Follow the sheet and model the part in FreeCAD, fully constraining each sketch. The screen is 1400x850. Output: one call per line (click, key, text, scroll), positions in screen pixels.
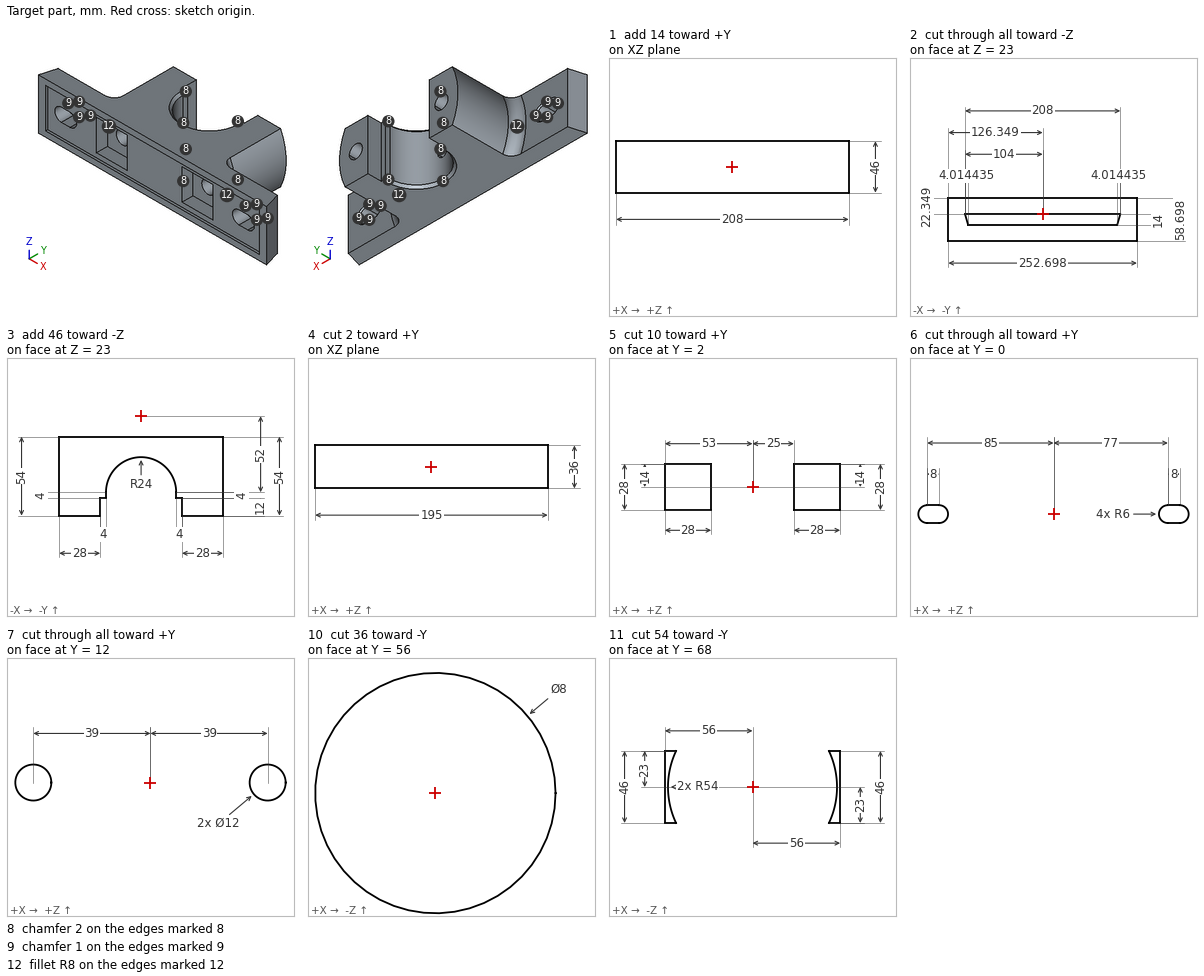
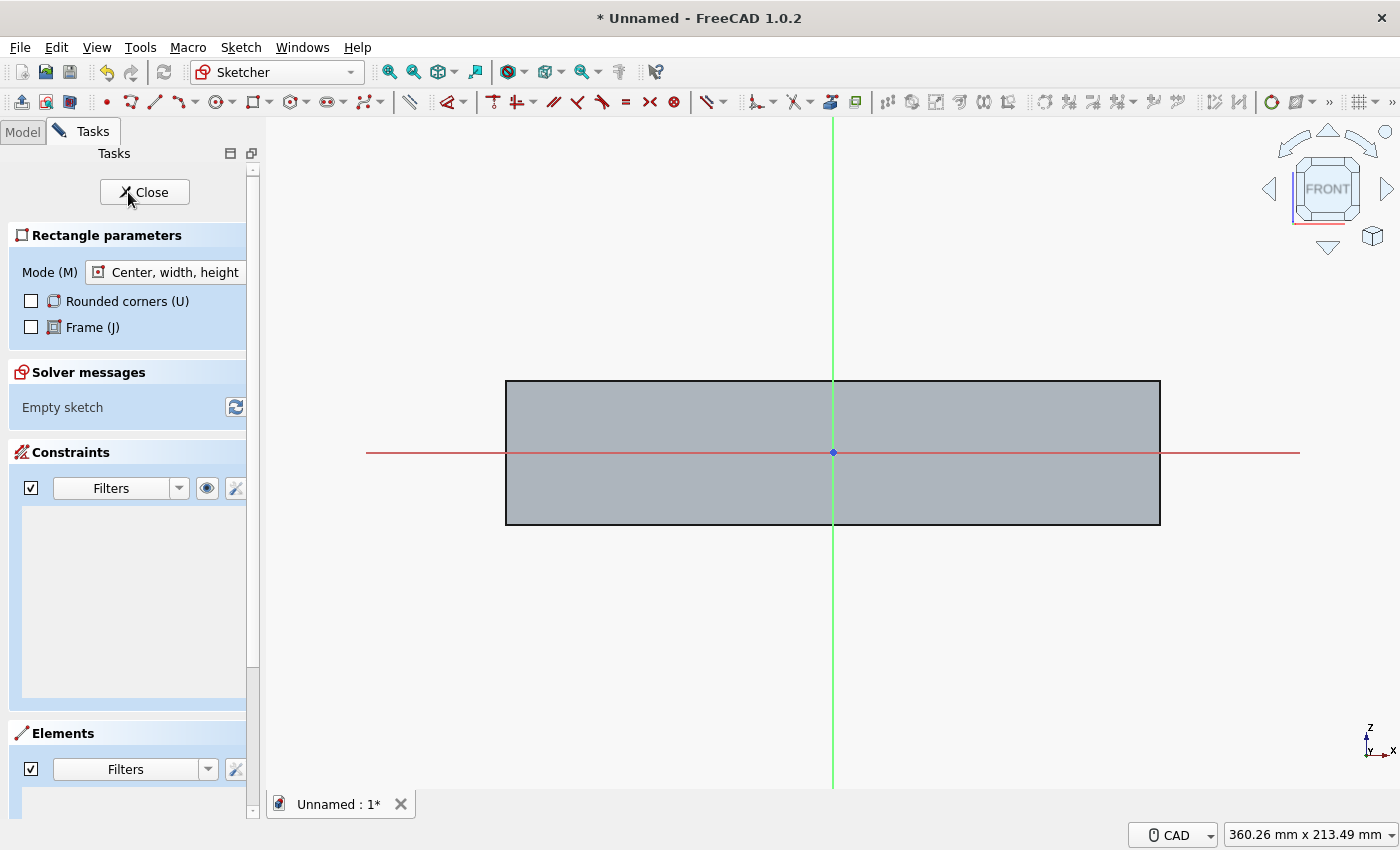
click(833, 453)
move(1140, 396)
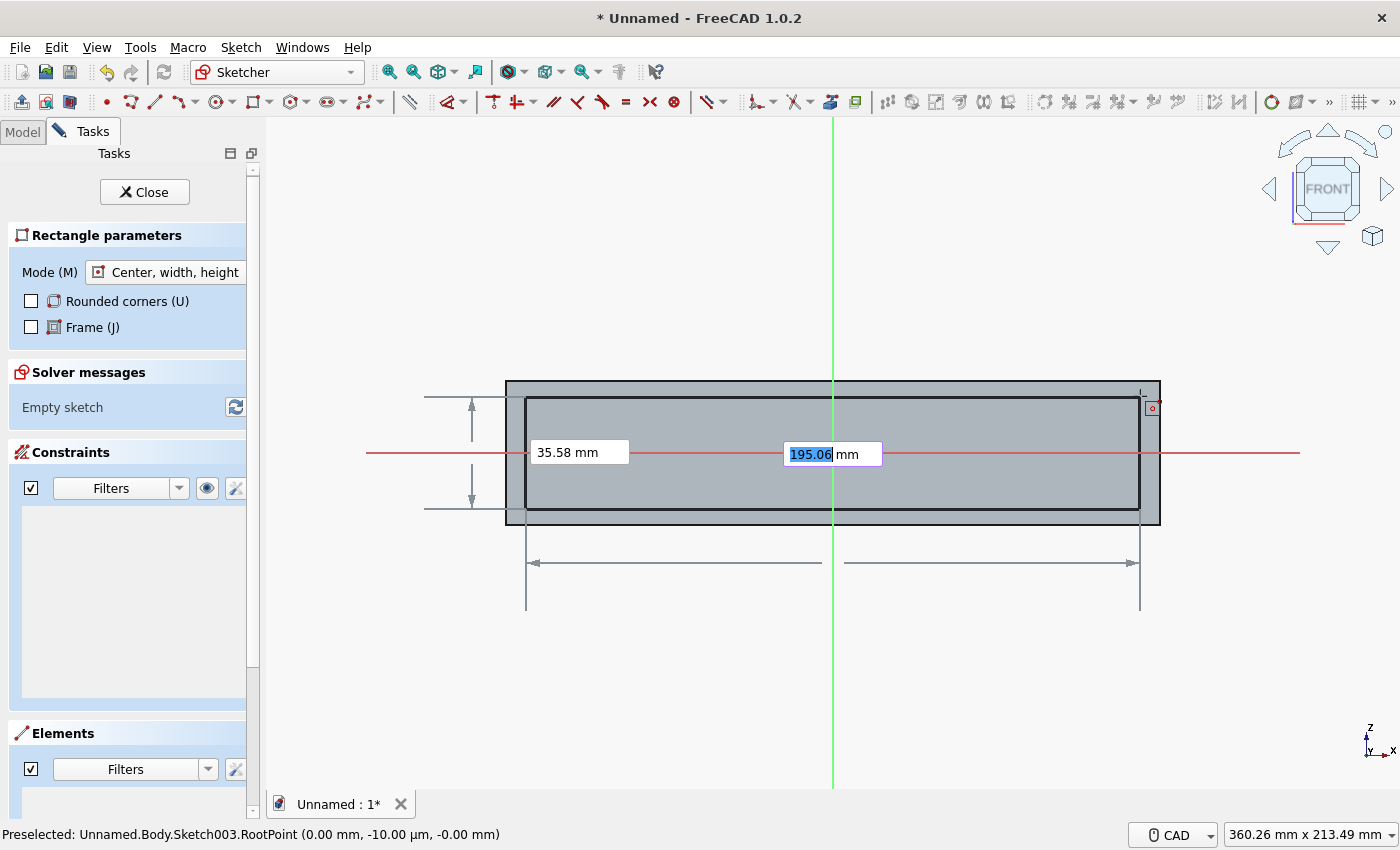
text(195)
key(Tab)
text(36)
key(Return)
key(Escape)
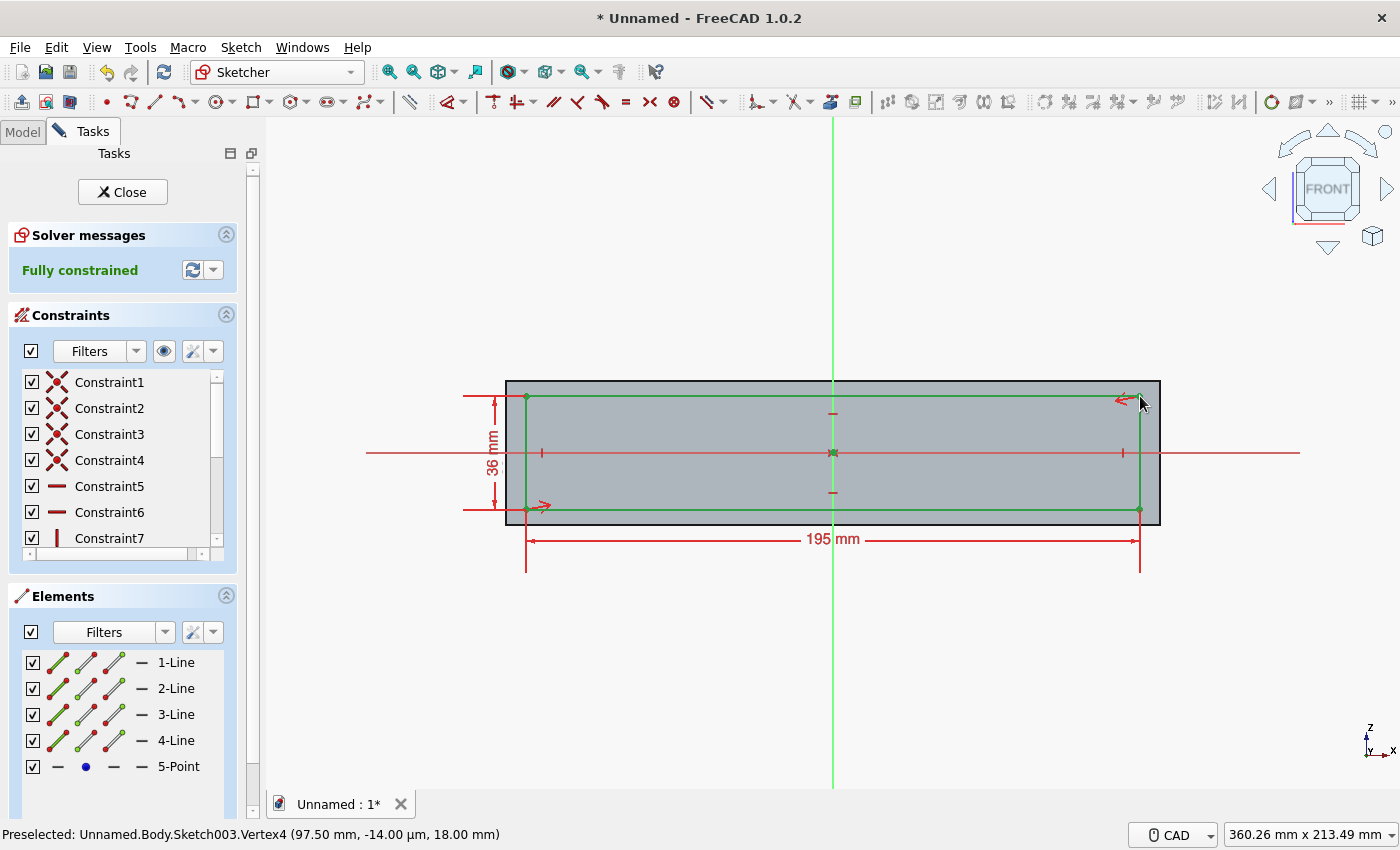
click(123, 192)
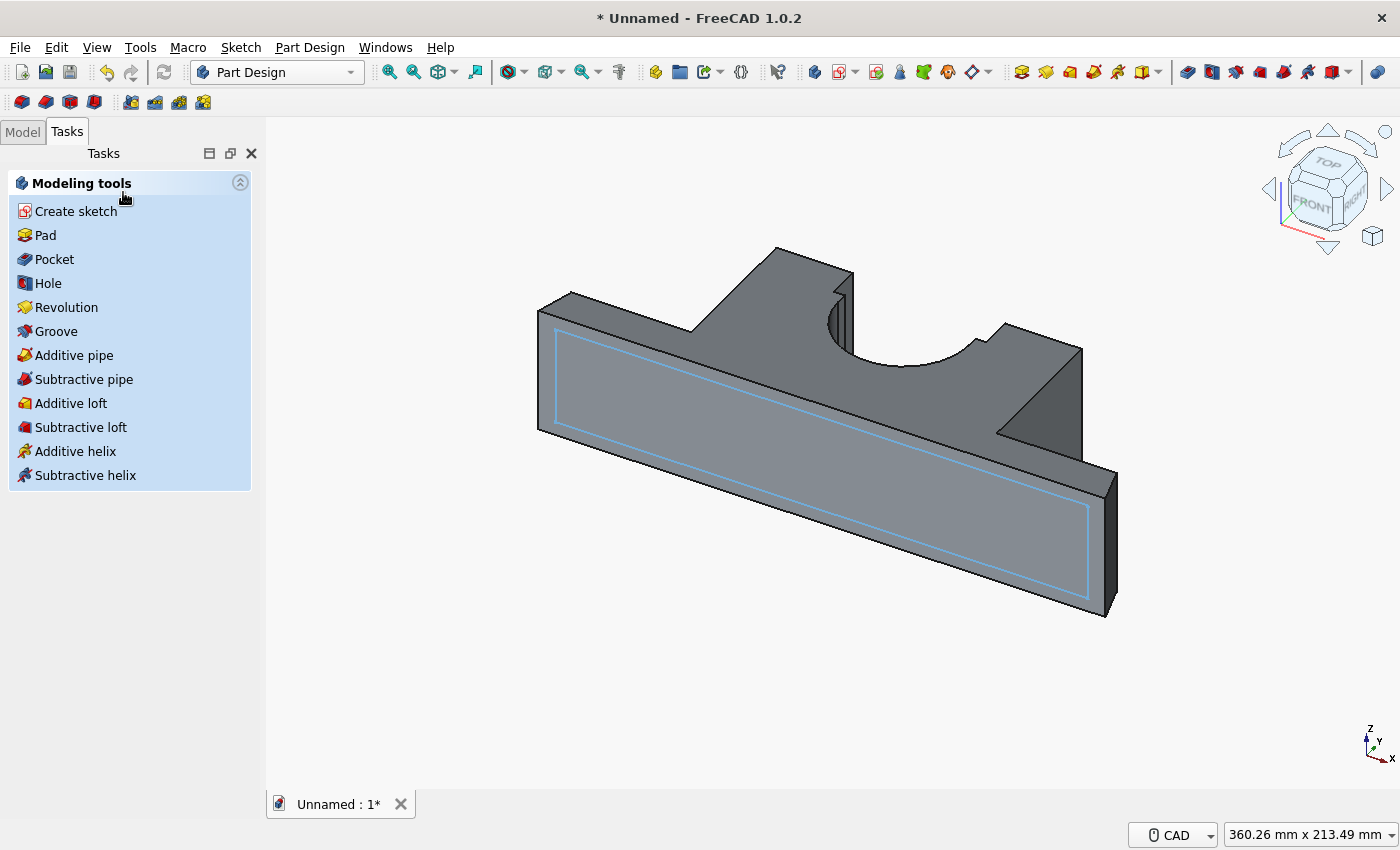
click(1188, 72)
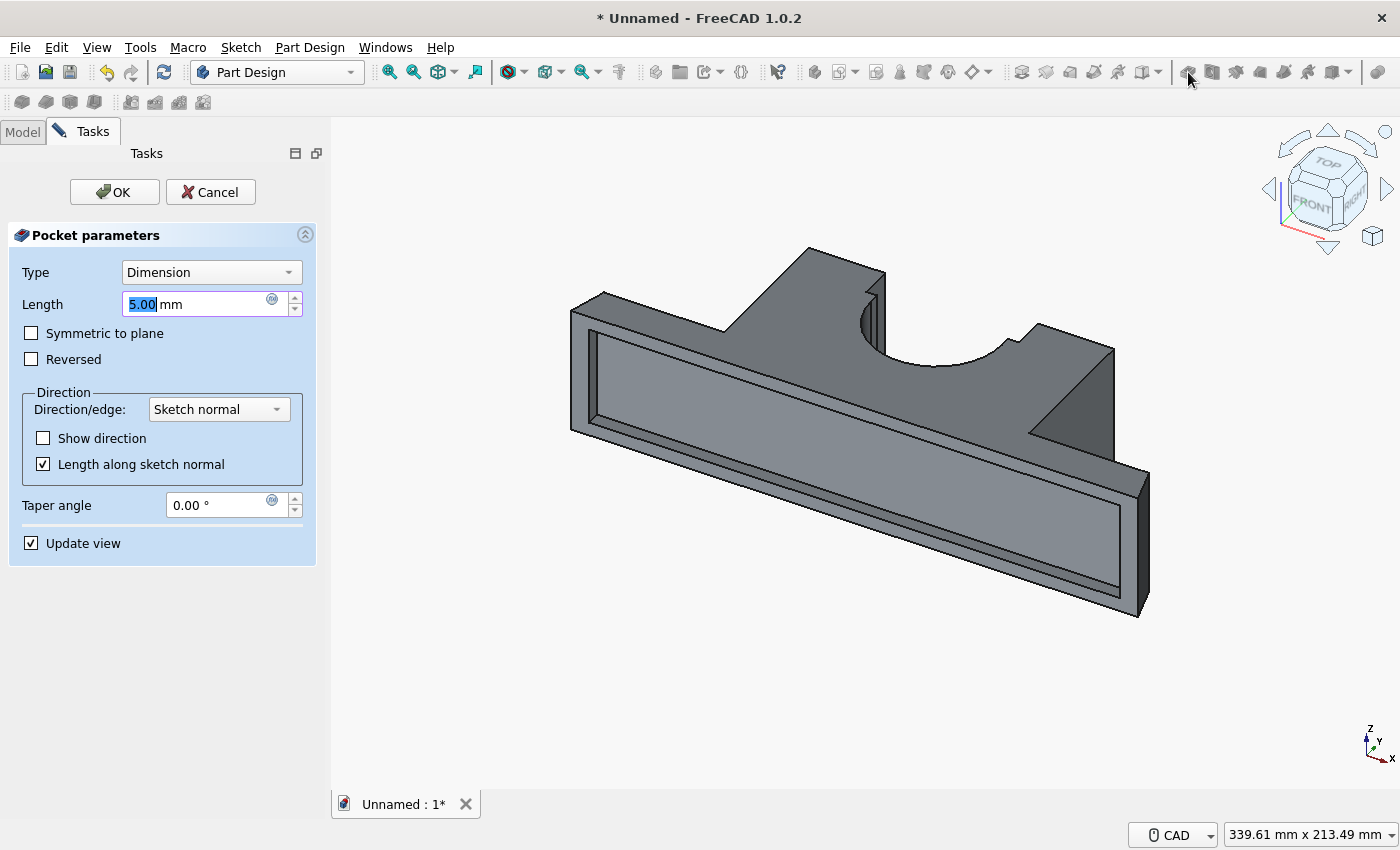
text(2)
key(Tab)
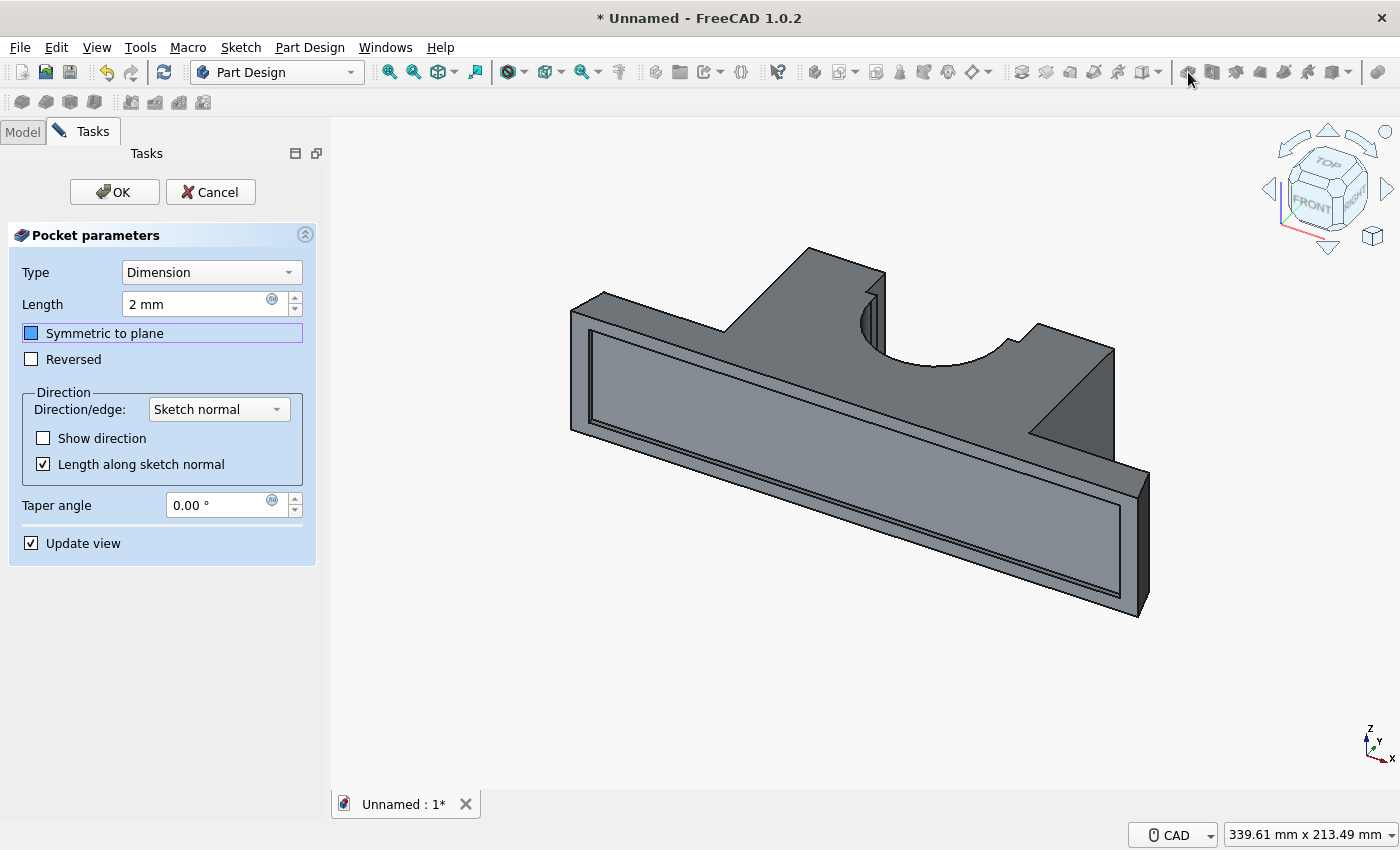
click(115, 192)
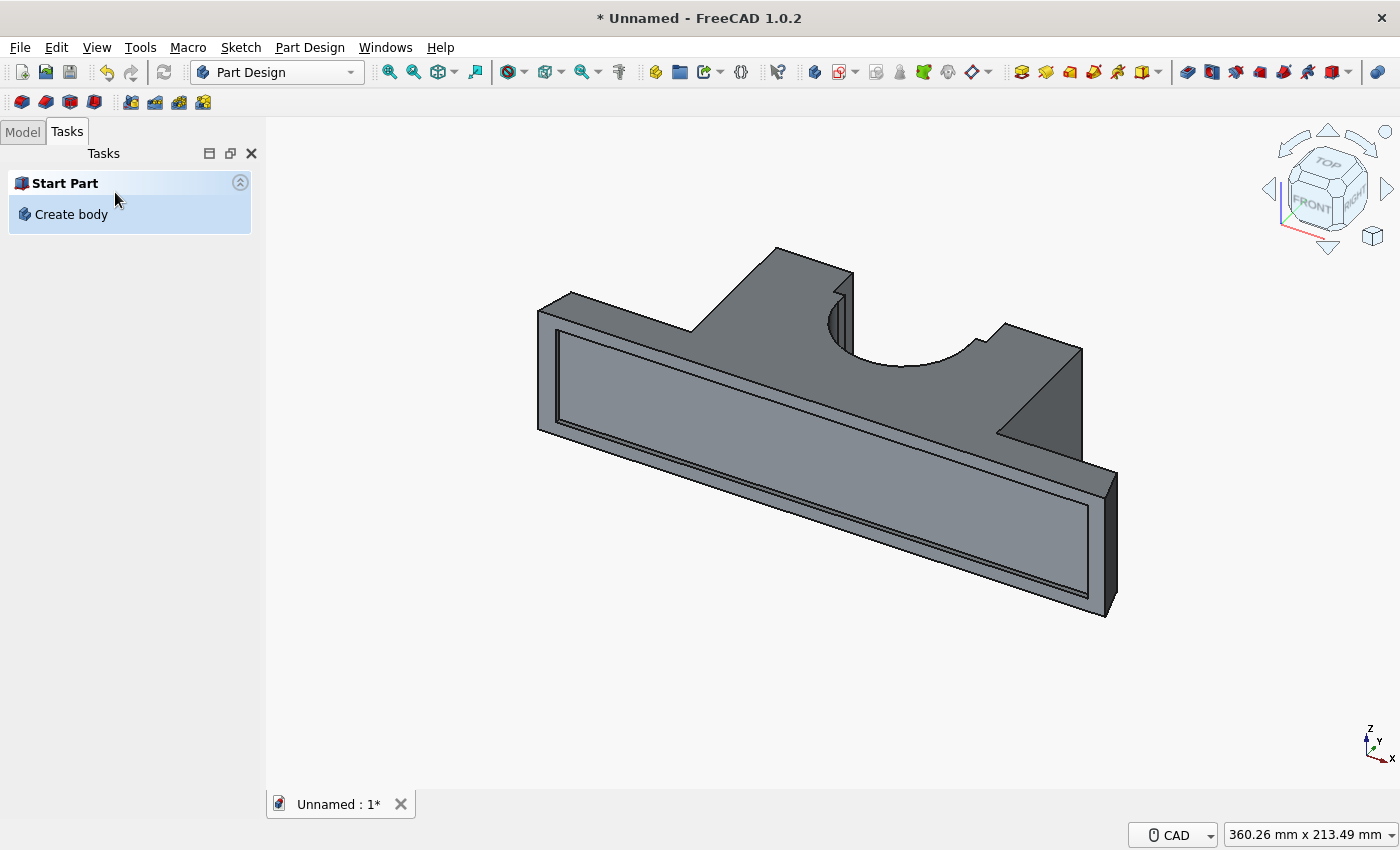
click(977, 510)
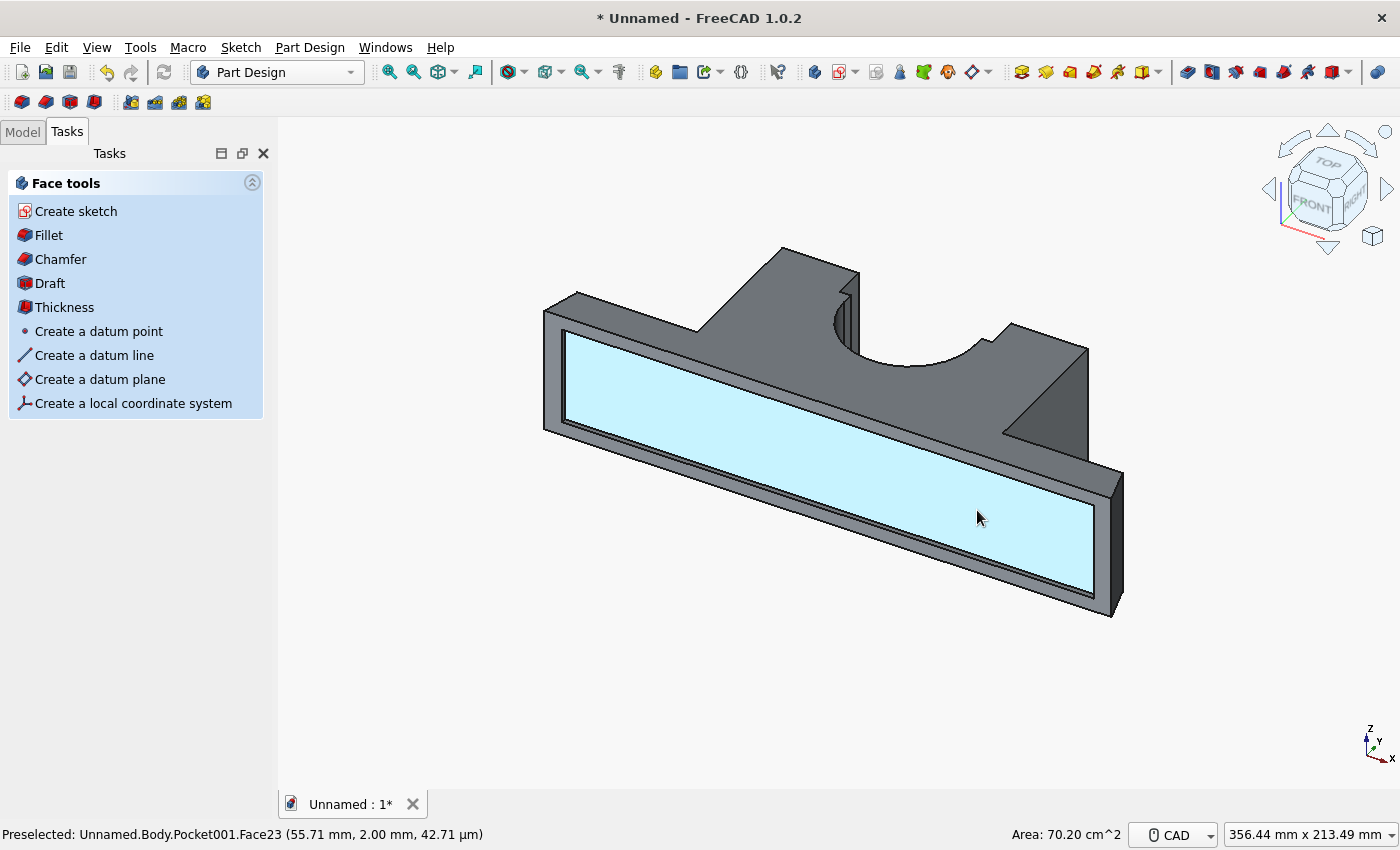
click(840, 72)